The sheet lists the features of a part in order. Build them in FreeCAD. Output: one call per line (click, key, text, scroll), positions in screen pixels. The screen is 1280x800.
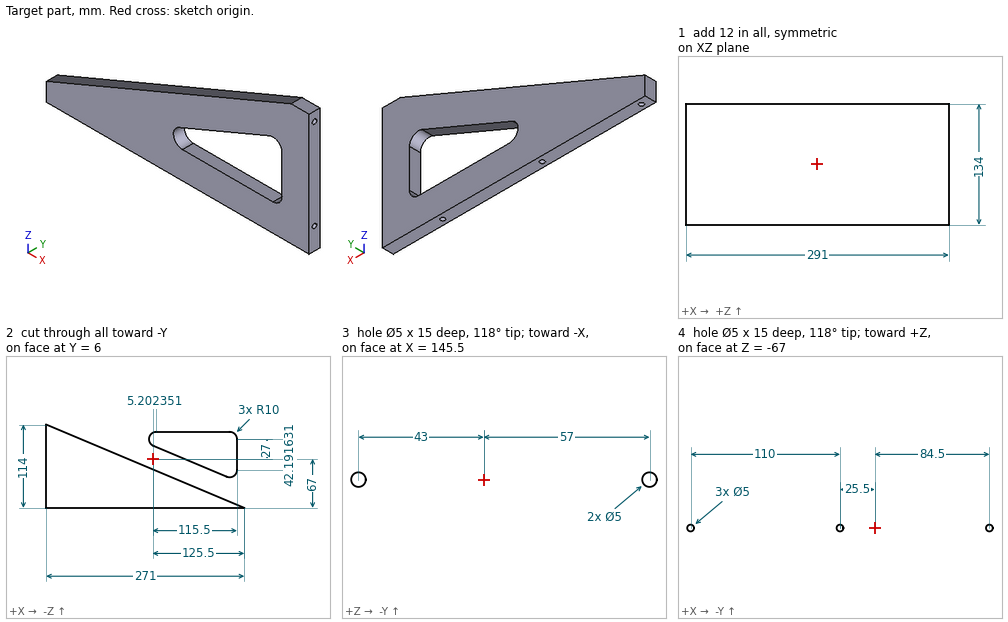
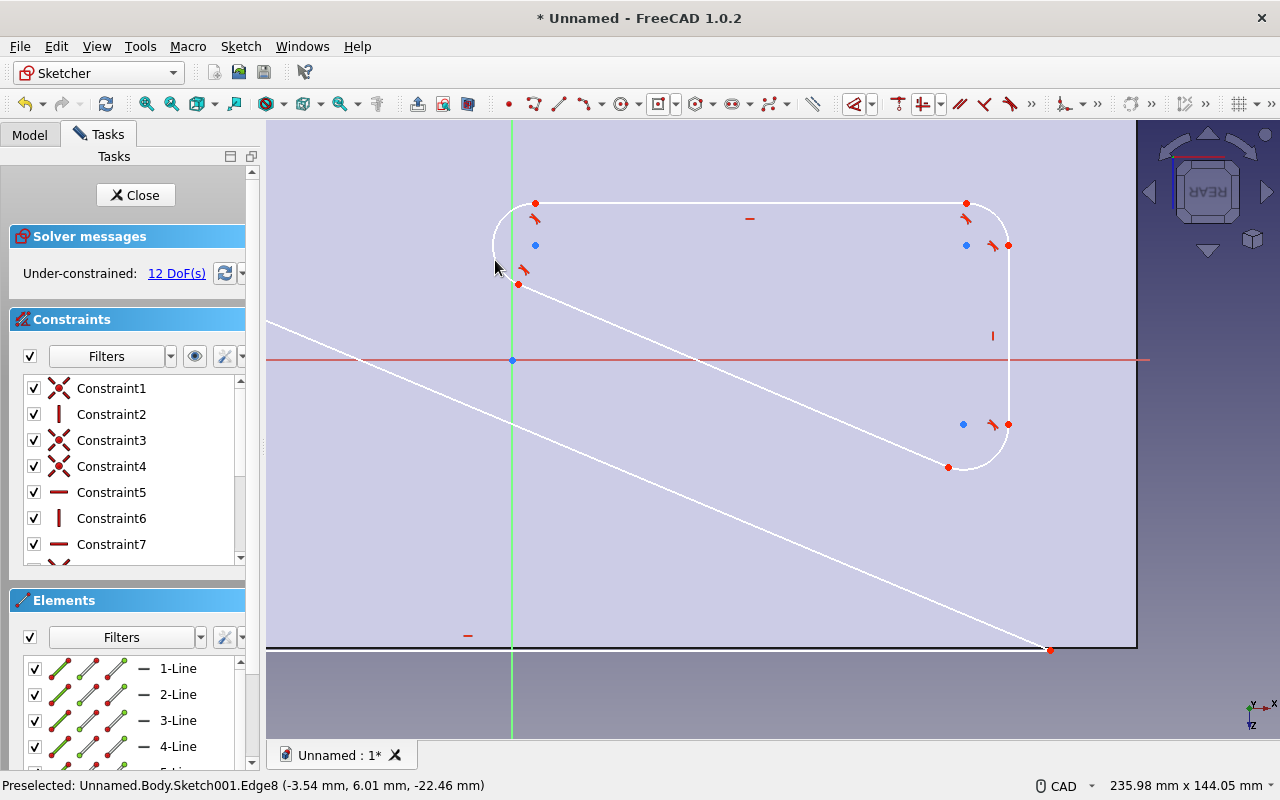
click(648, 339)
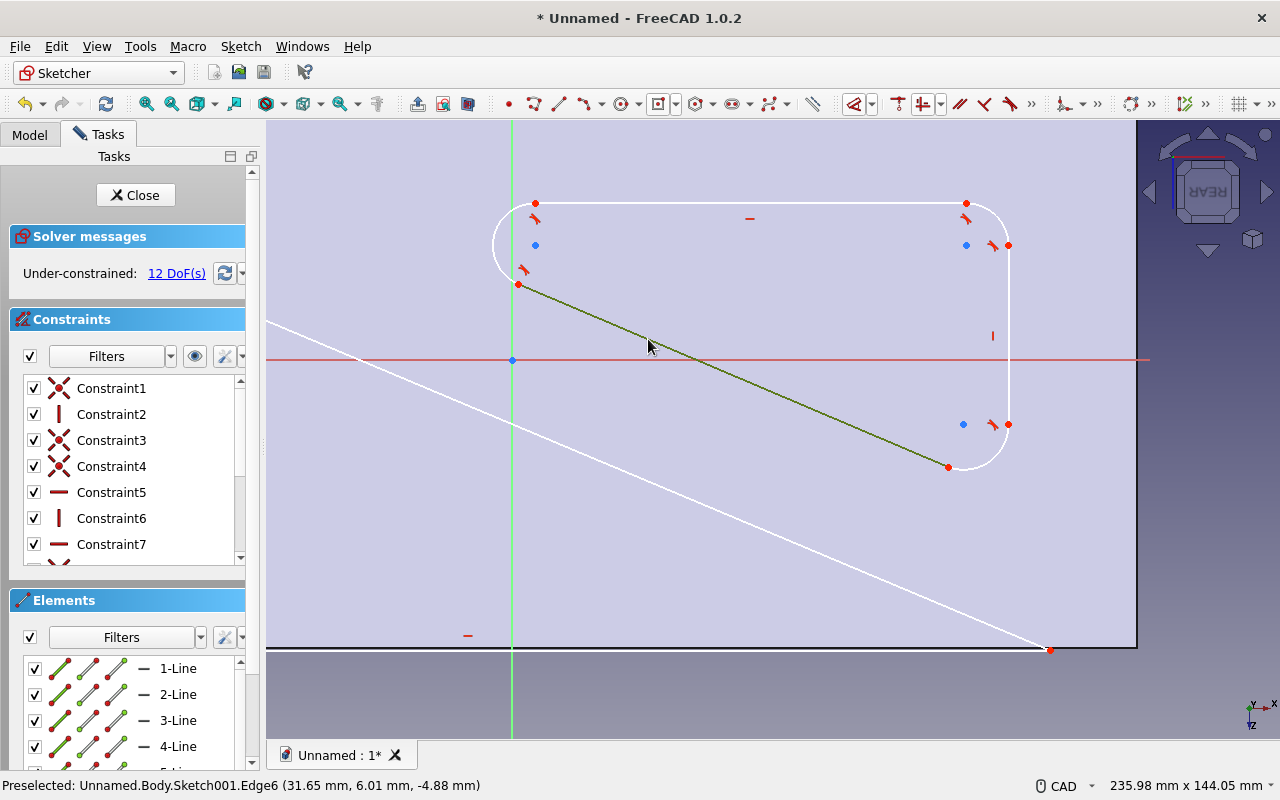
click(974, 469)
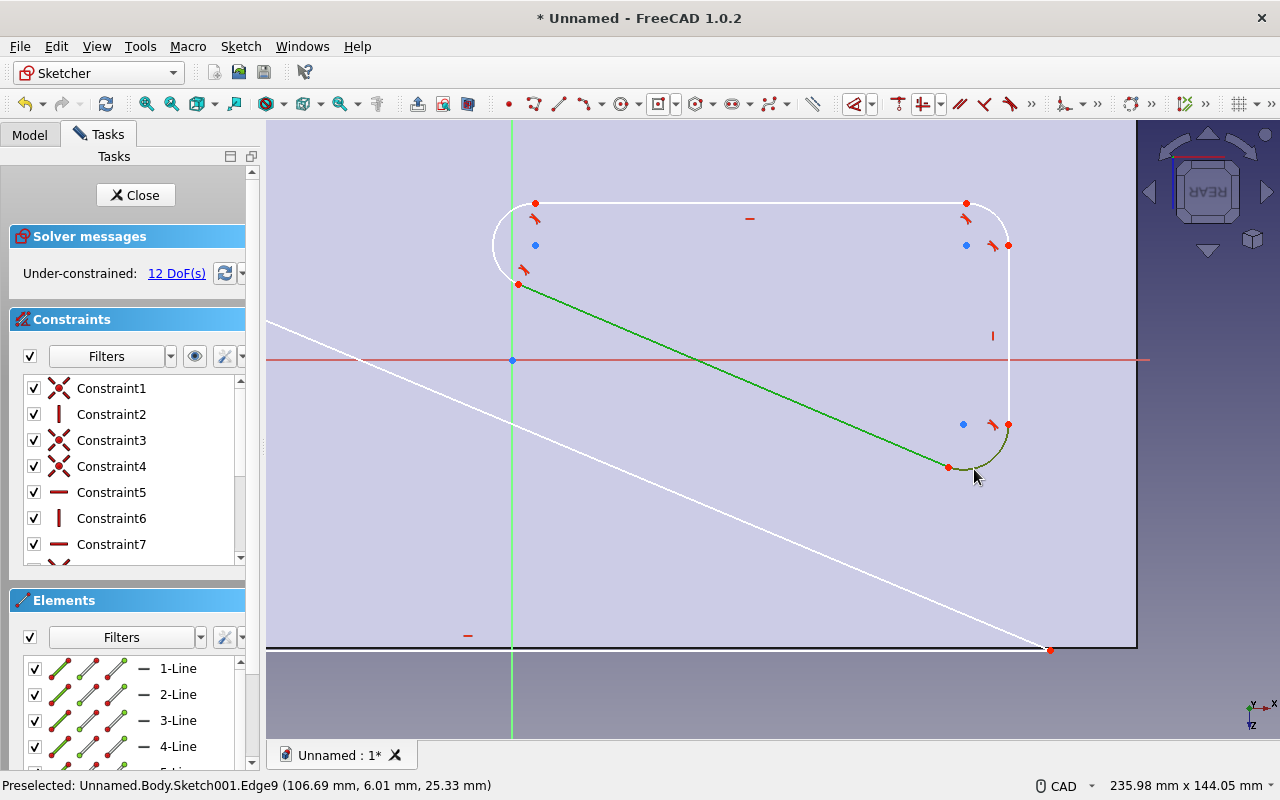
click(1010, 104)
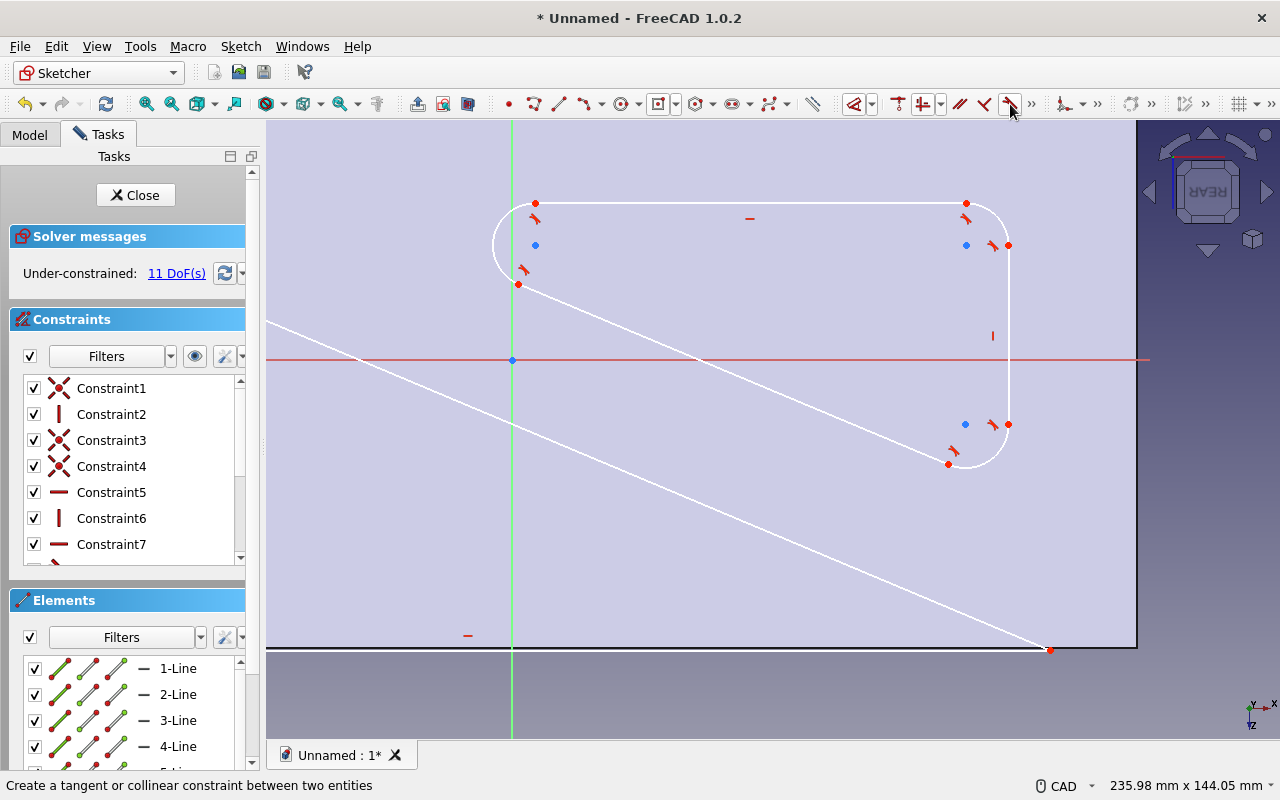
click(1004, 227)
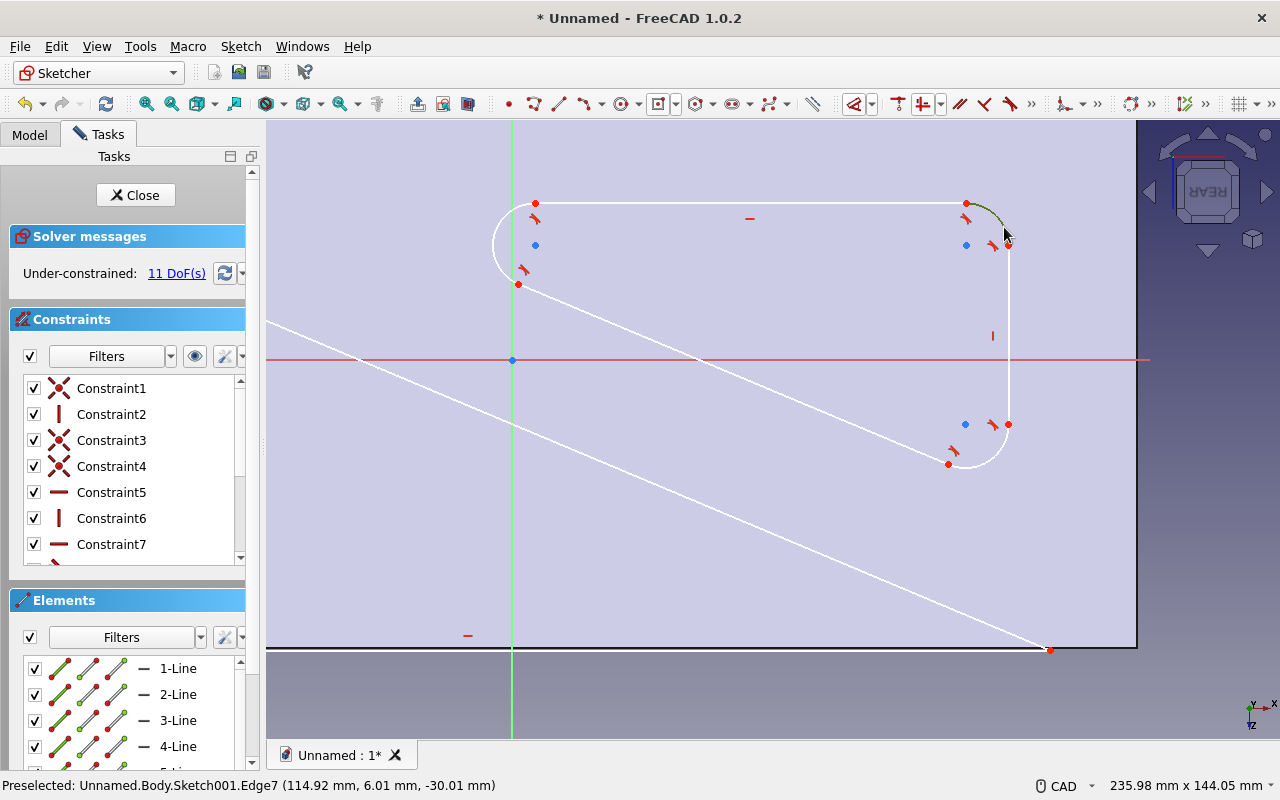
click(496, 260)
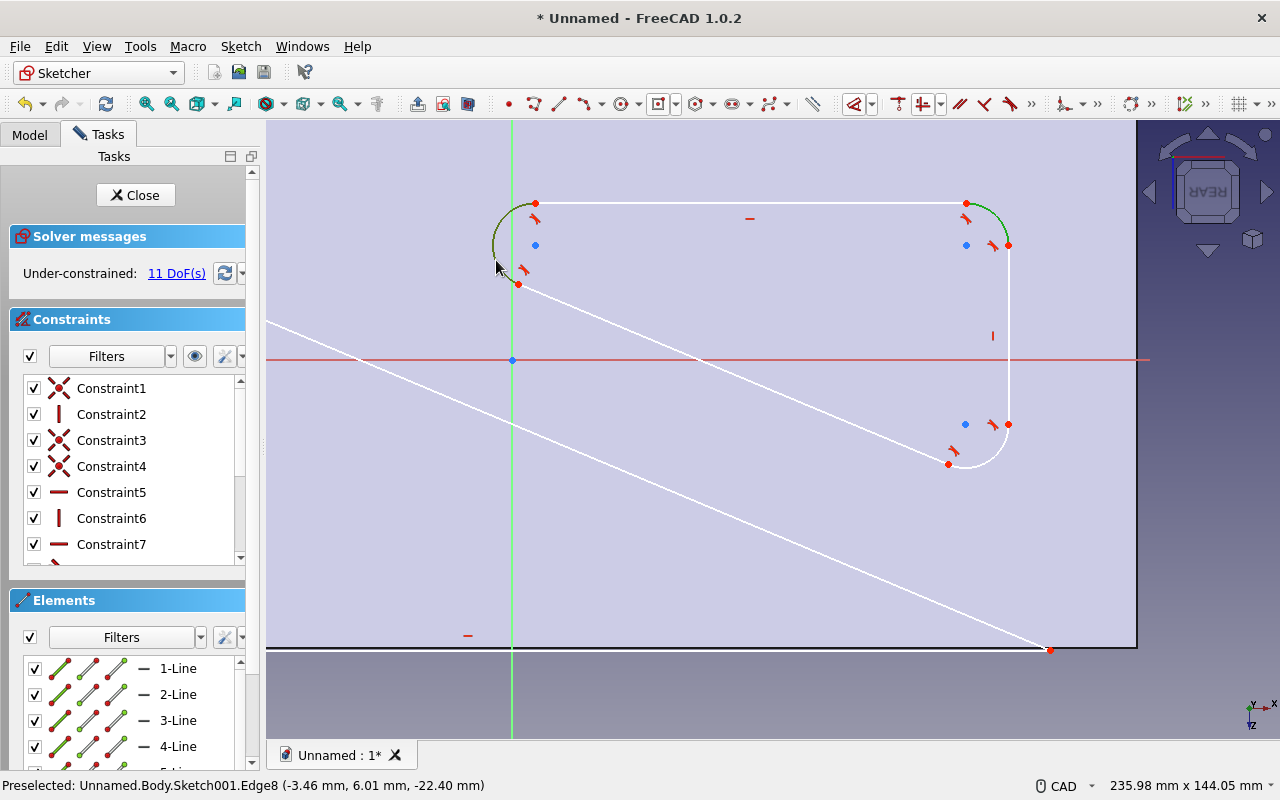
click(974, 467)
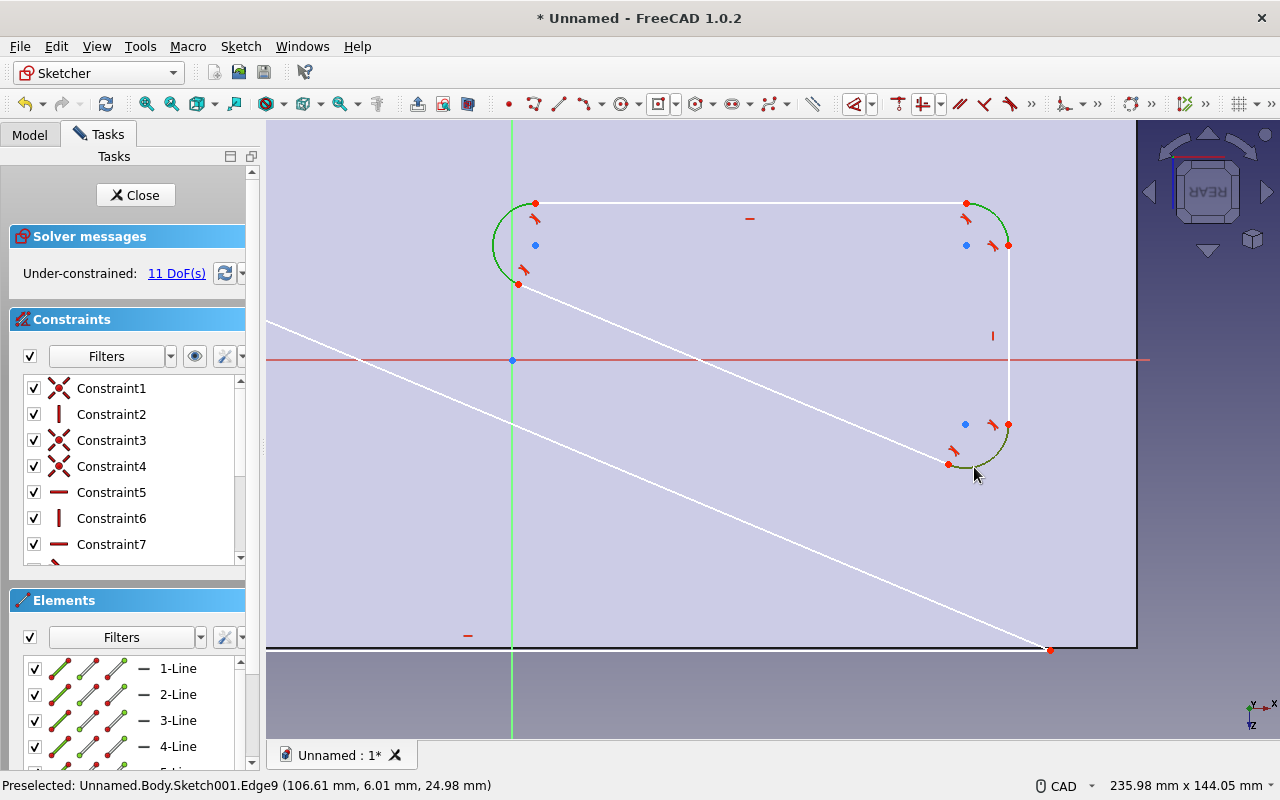
key(e)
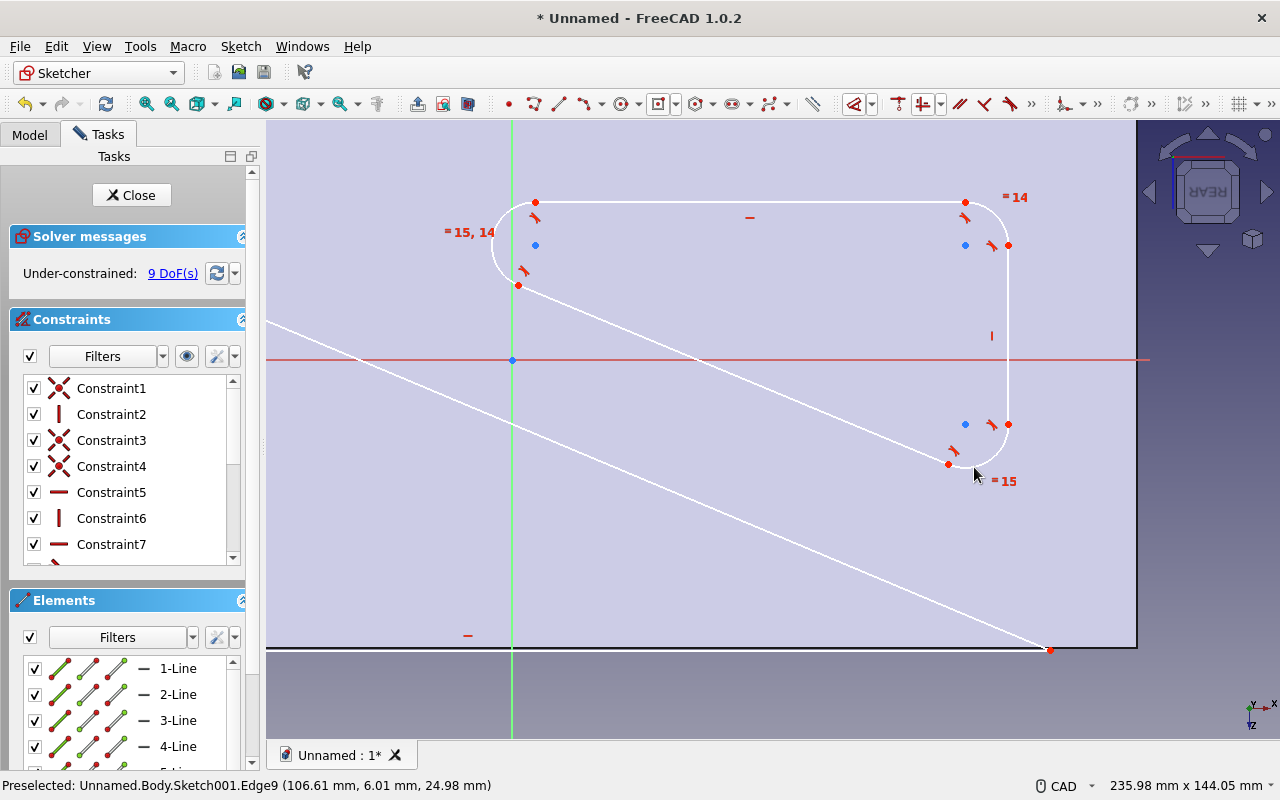
key(d)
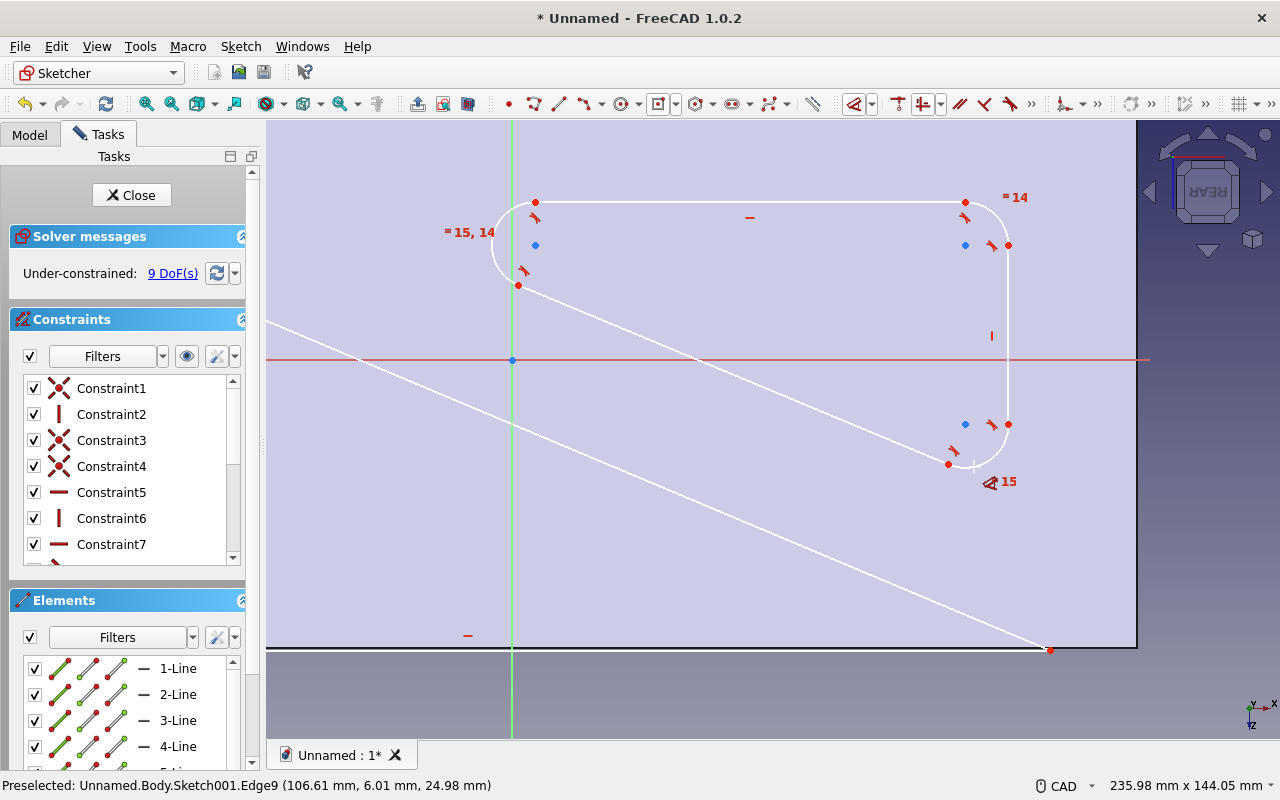
click(1004, 226)
click(1033, 212)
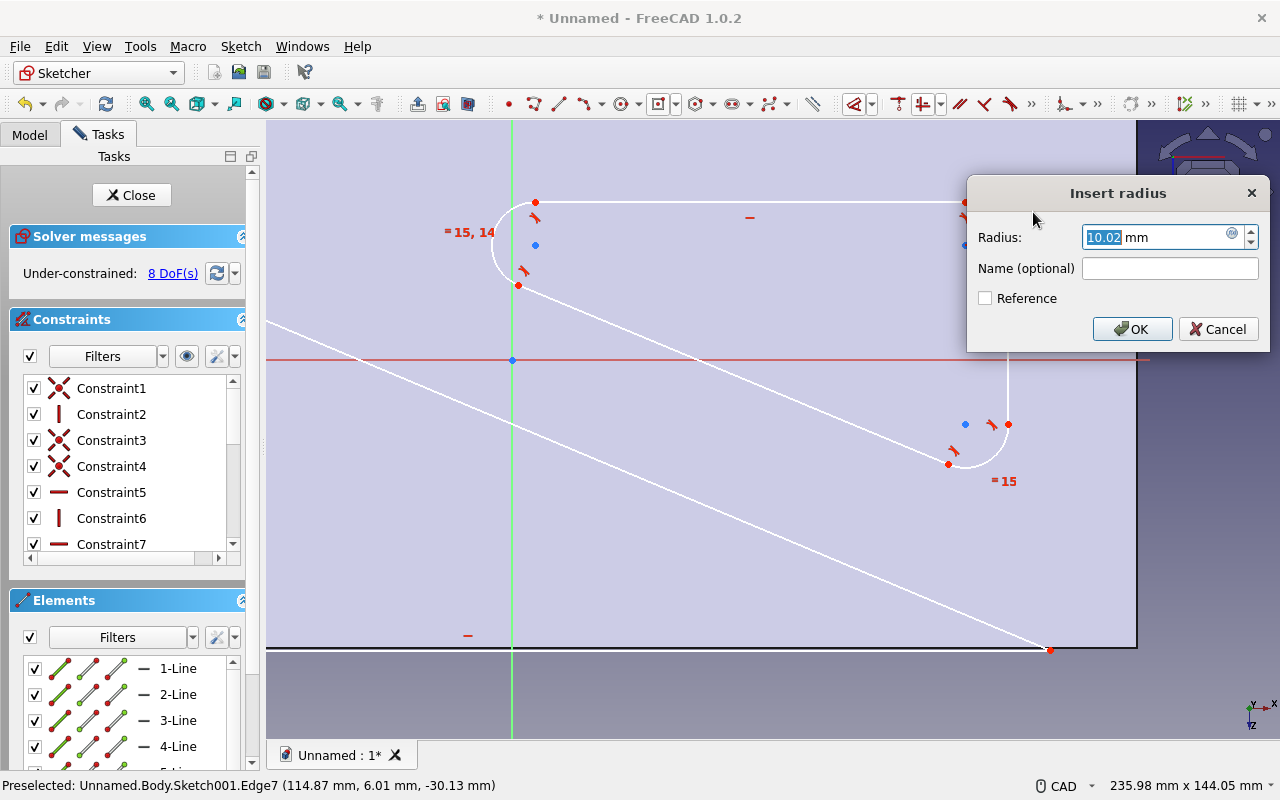
text(10)
key(Return)